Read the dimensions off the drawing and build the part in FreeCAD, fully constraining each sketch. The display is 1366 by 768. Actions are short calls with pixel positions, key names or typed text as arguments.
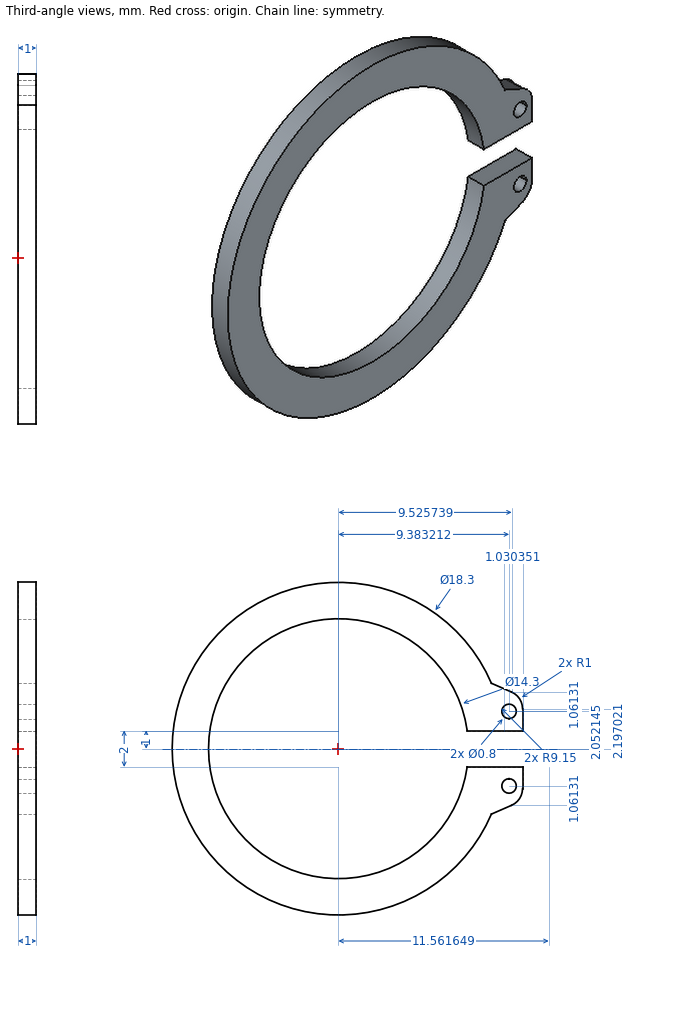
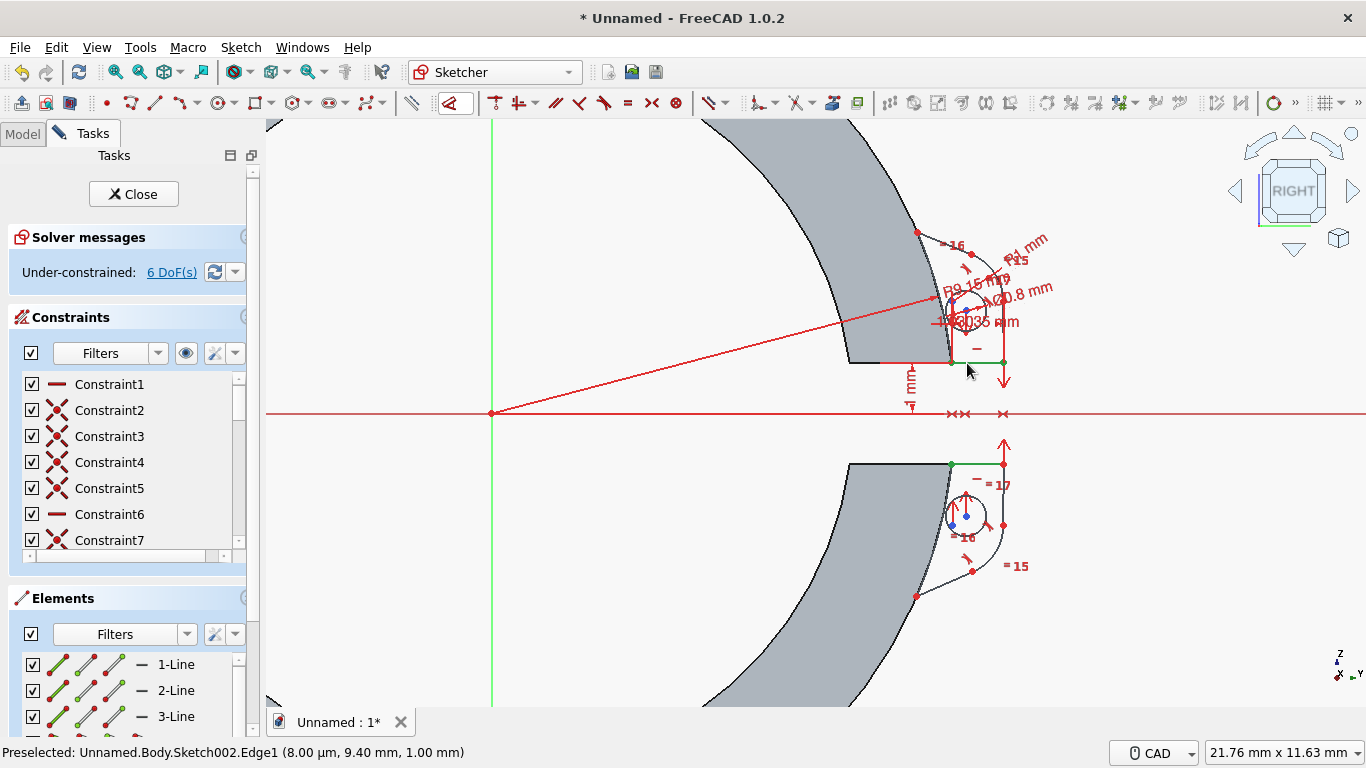
click(966, 311)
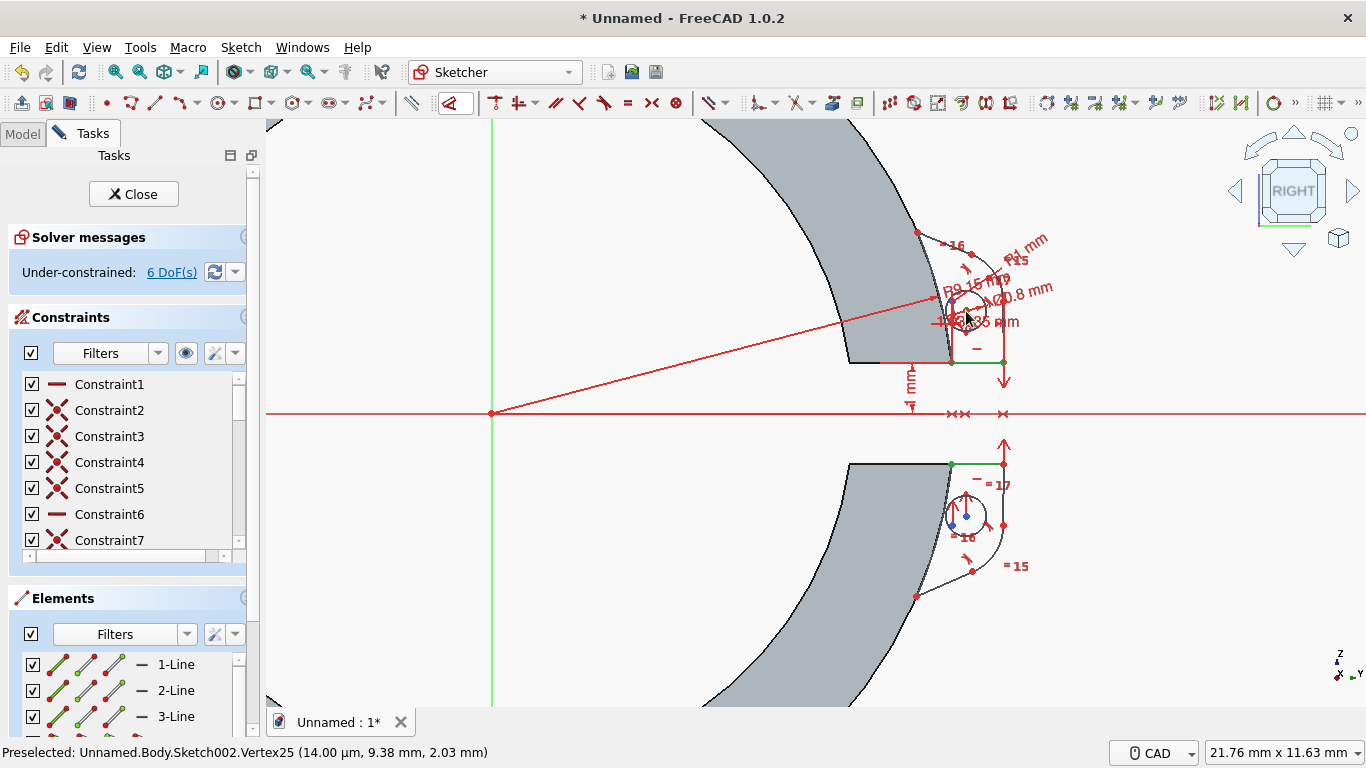
key(l)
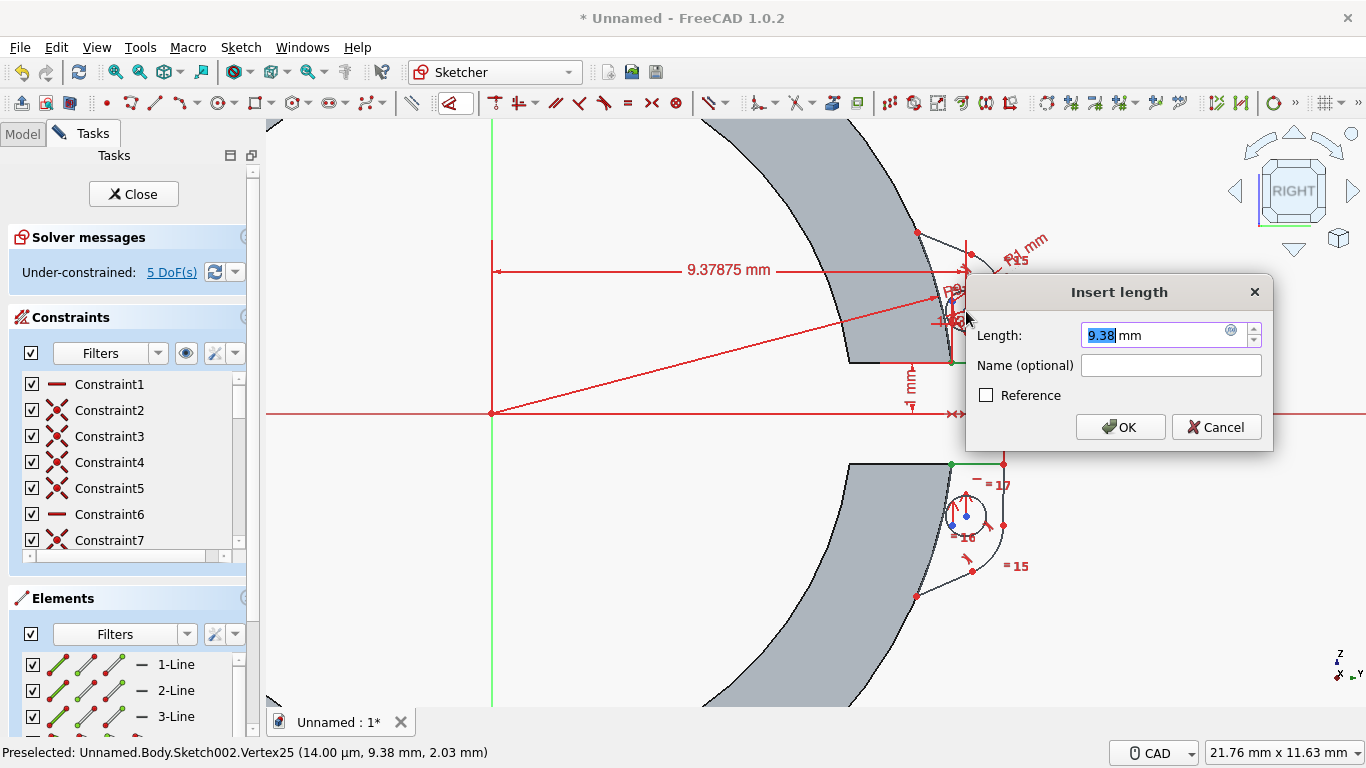
text(9.383212)
key(Return)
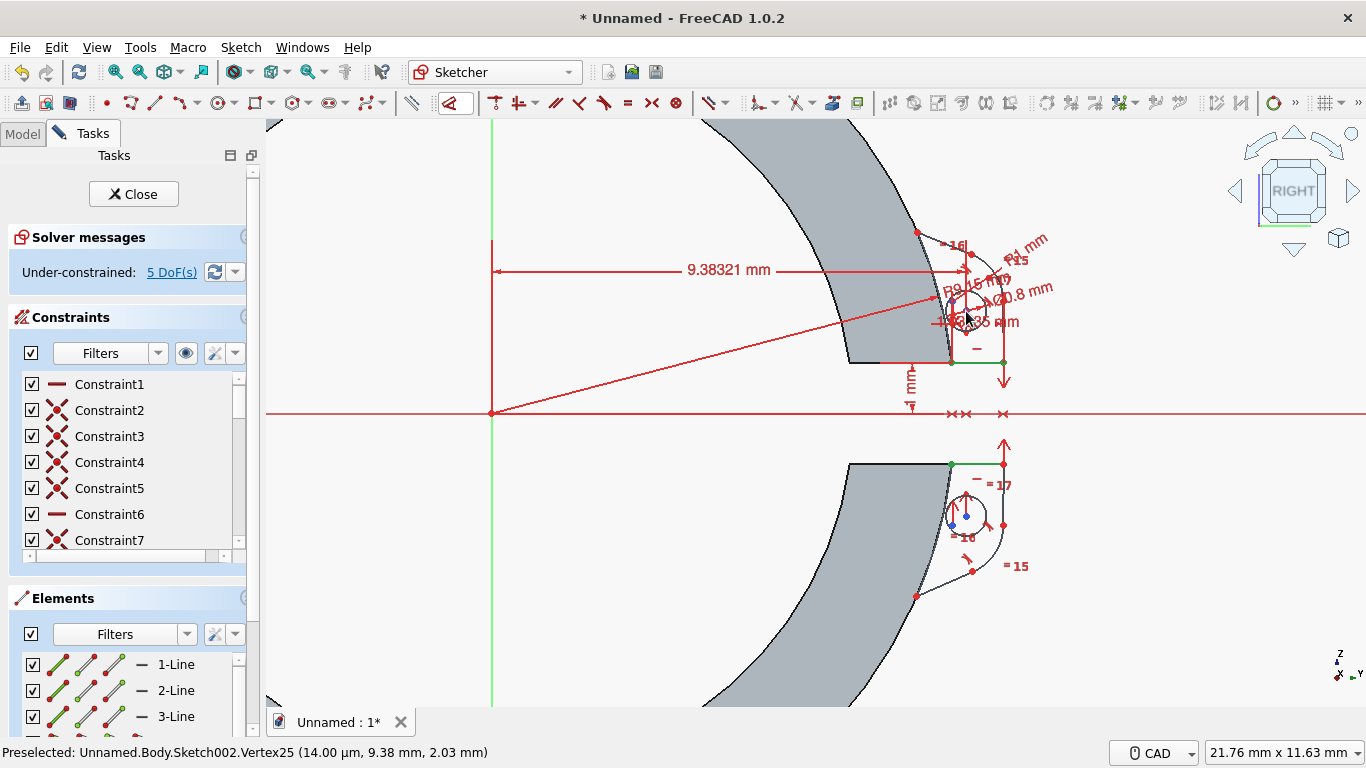
click(966, 311)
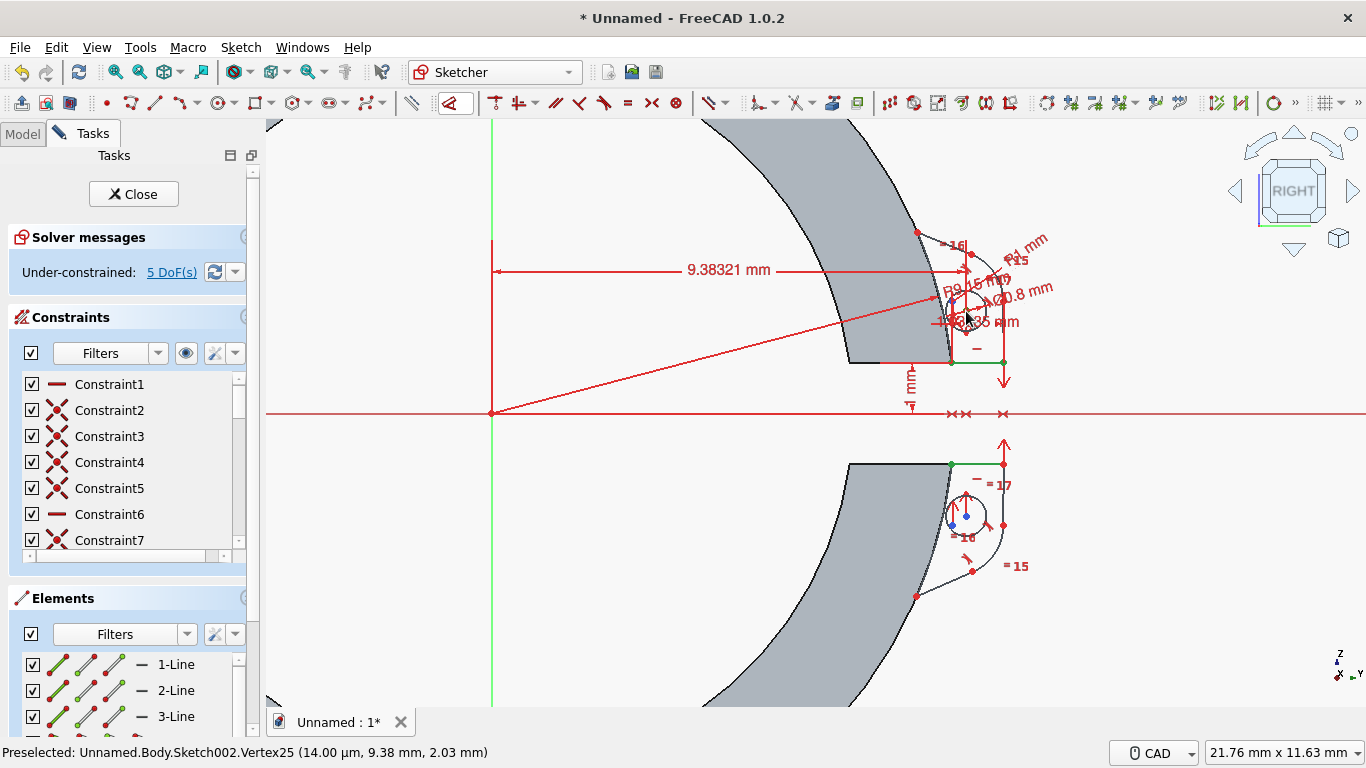
click(468, 104)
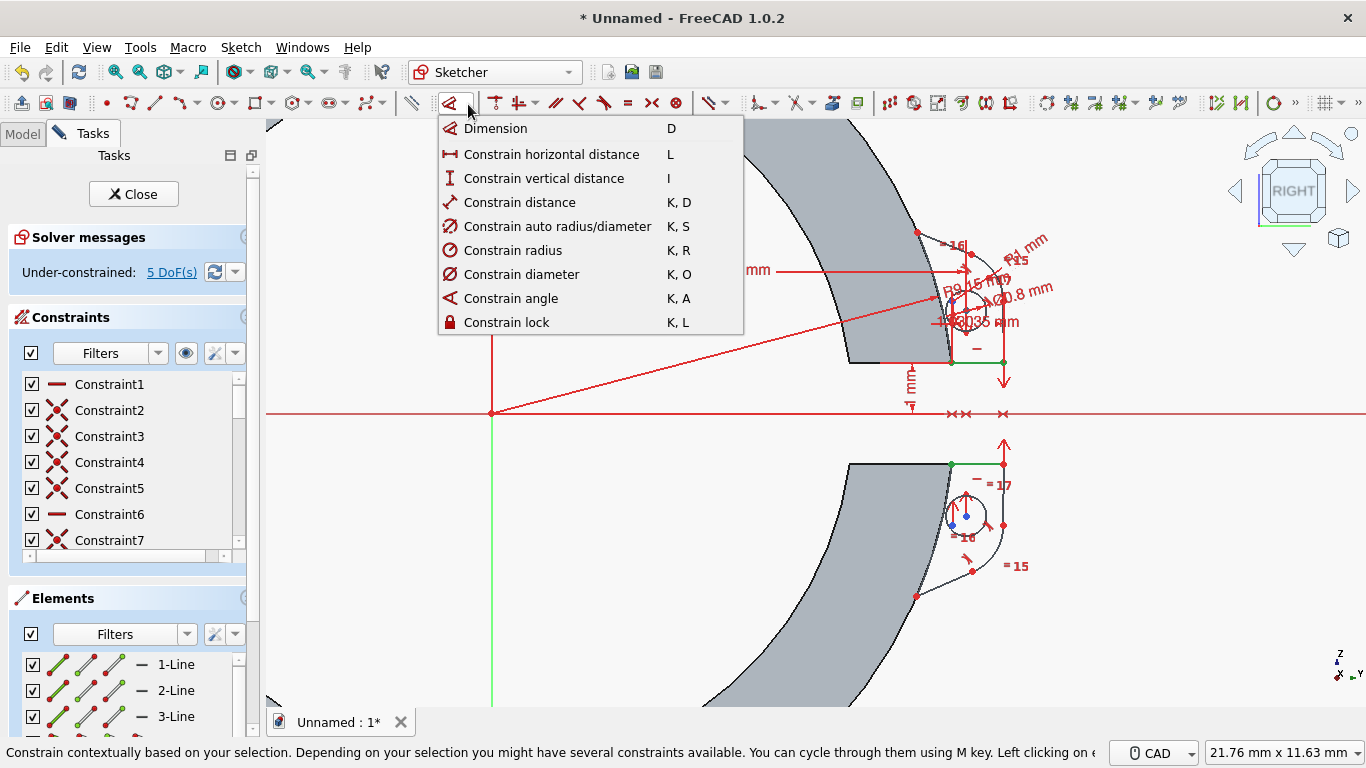
click(591, 178)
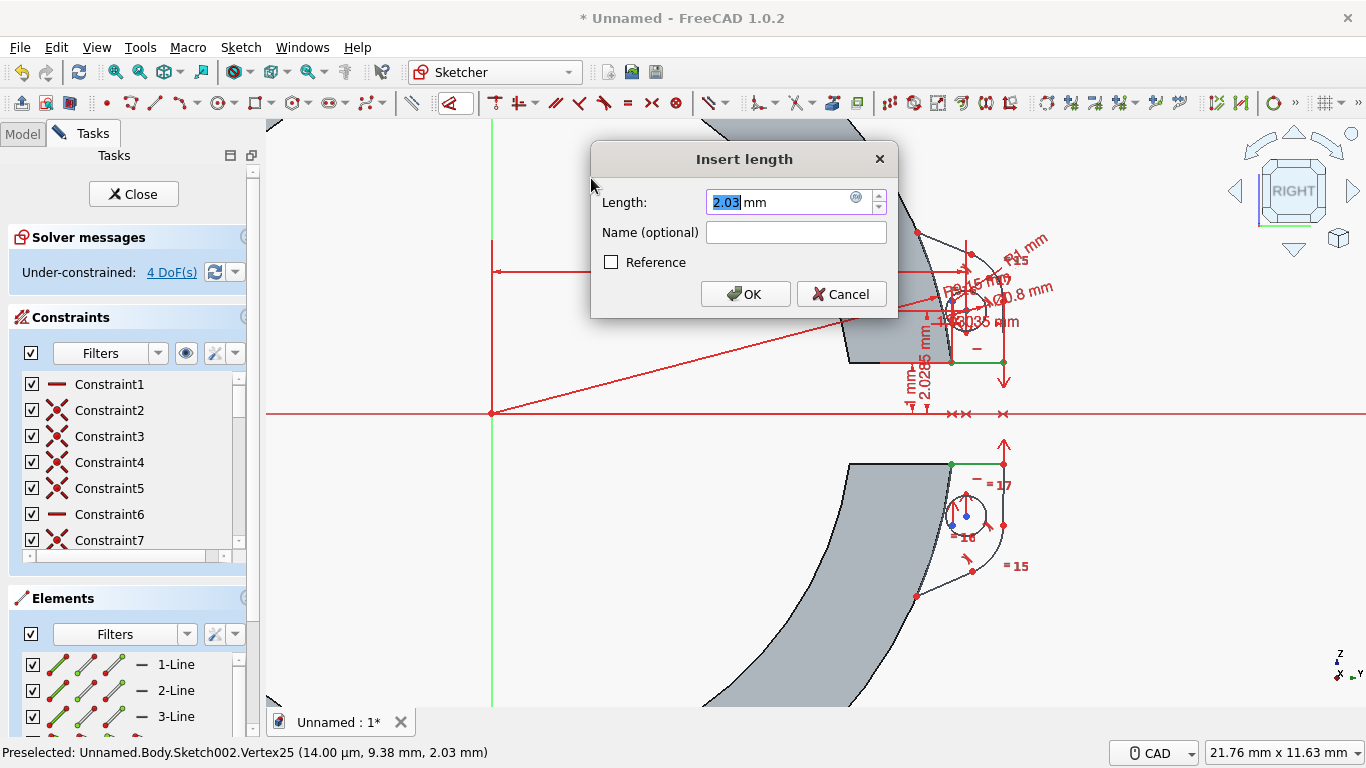
text(2.052145)
key(Return)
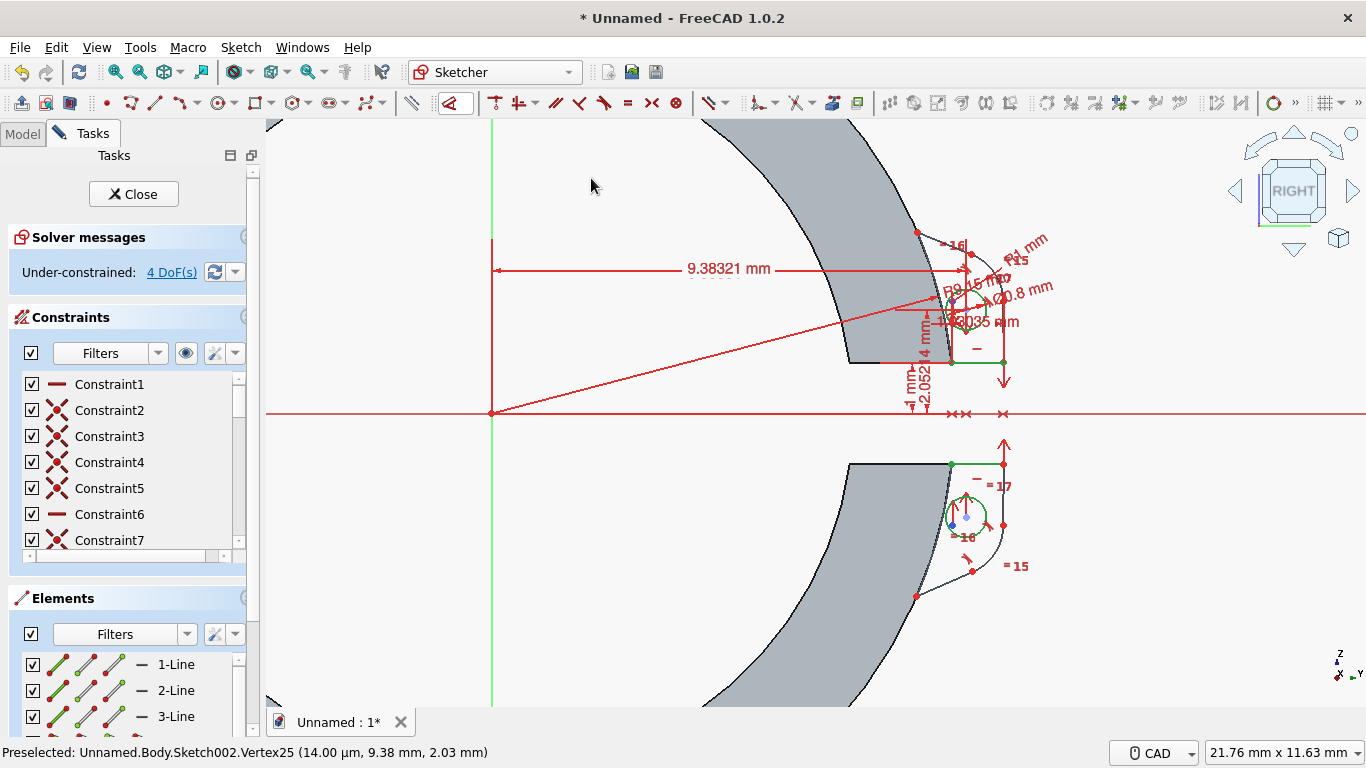
click(972, 255)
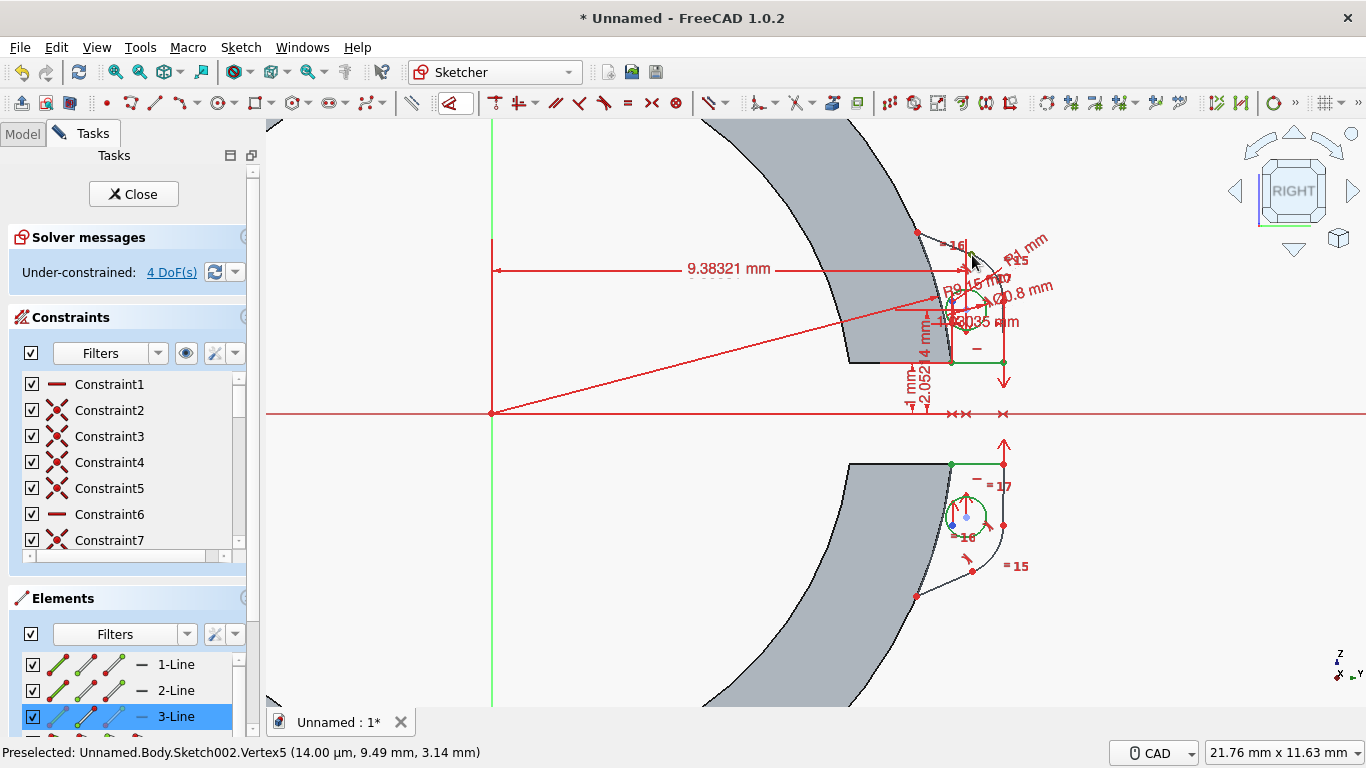
click(966, 310)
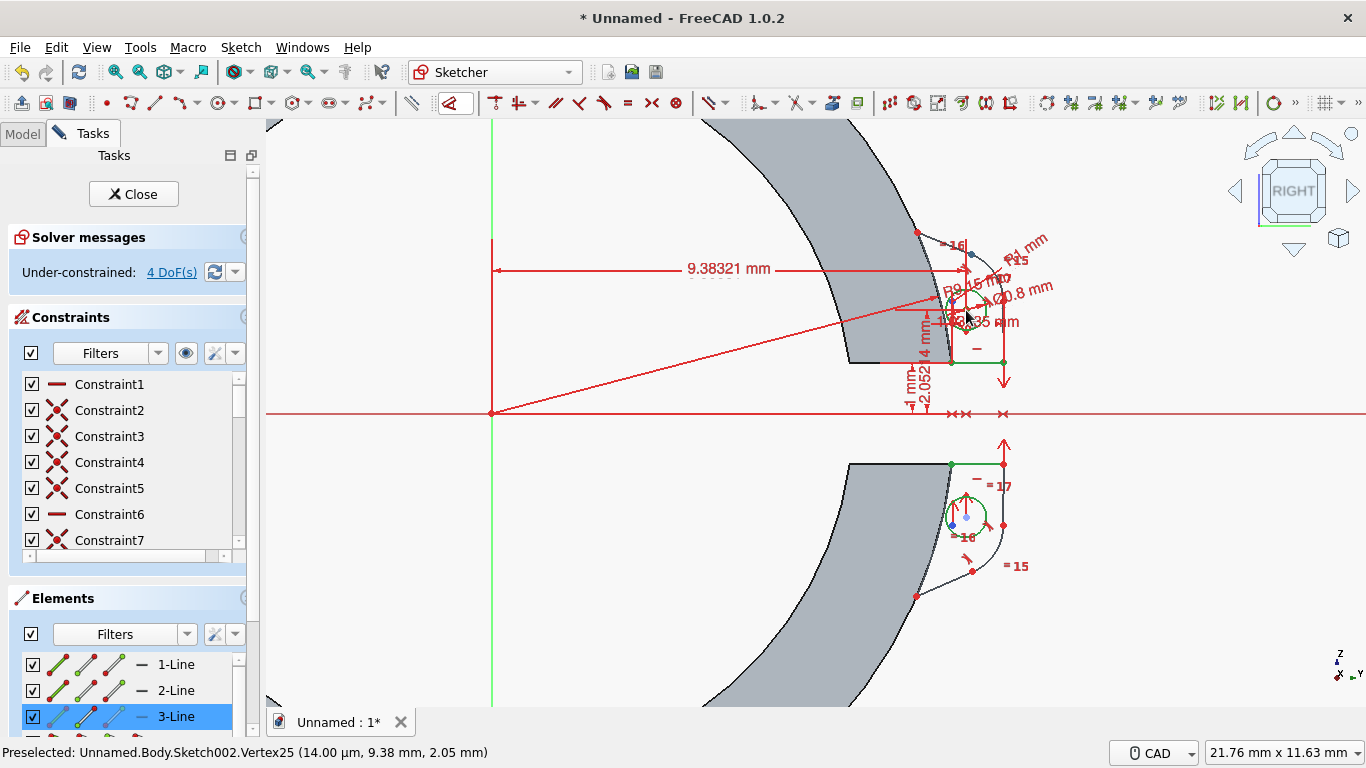
click(468, 104)